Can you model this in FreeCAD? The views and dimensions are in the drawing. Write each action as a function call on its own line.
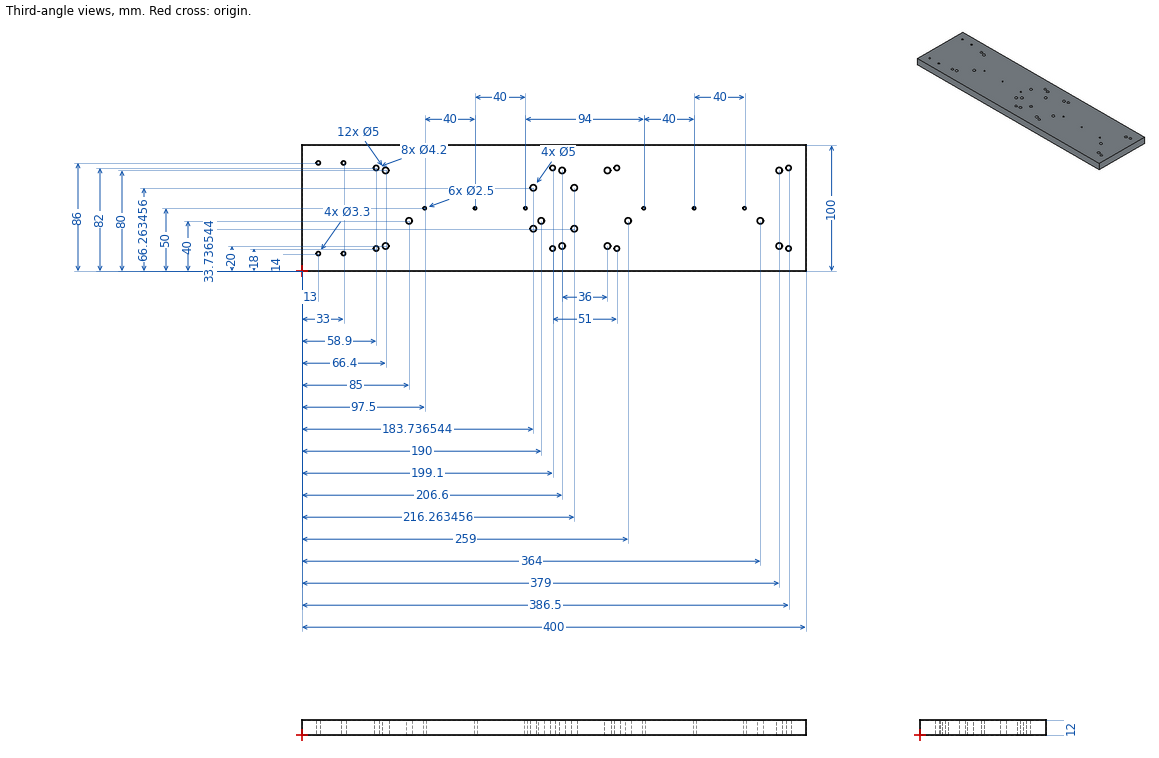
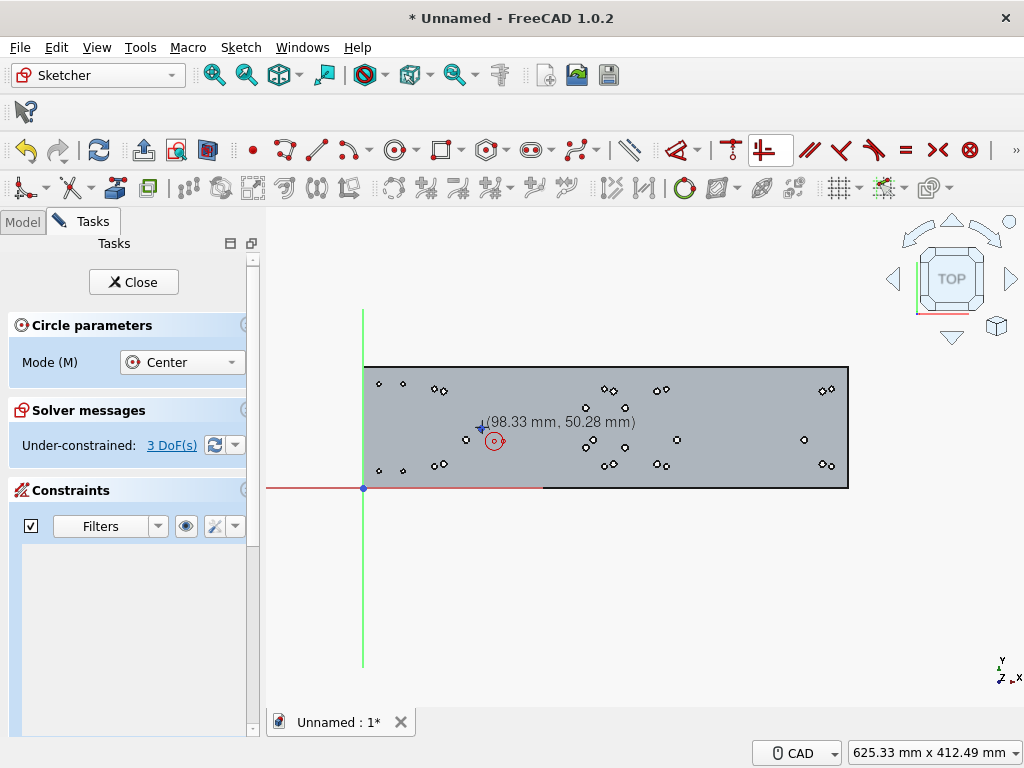
scroll(530, 428, up, 14)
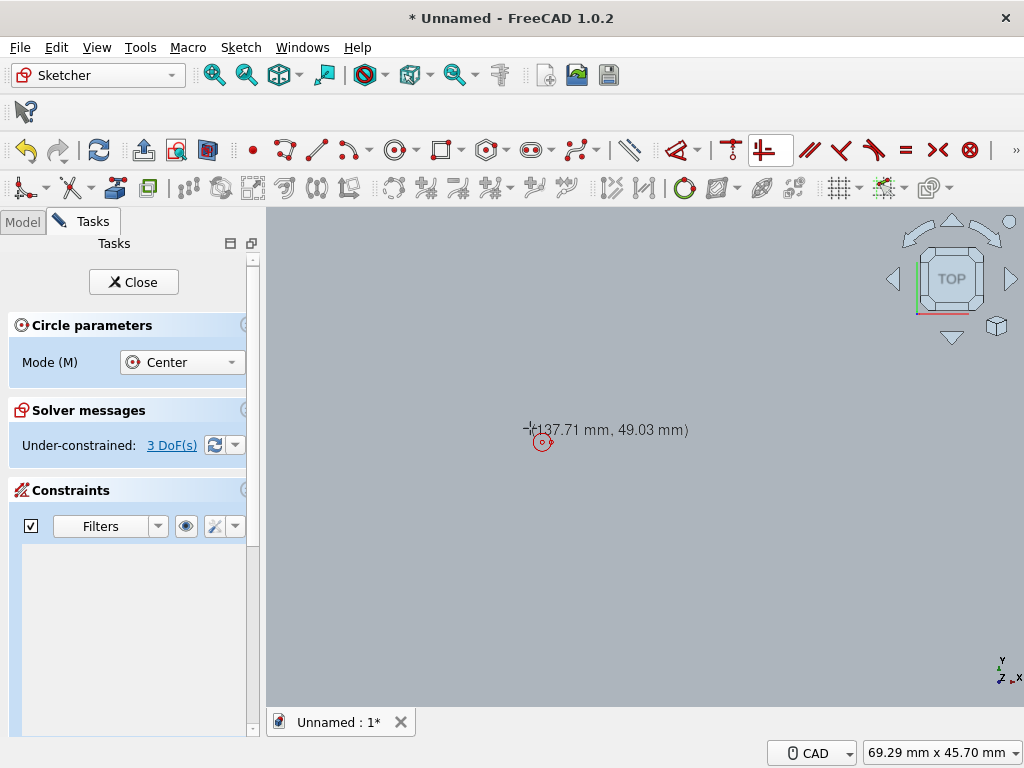
scroll(530, 428, down, 14)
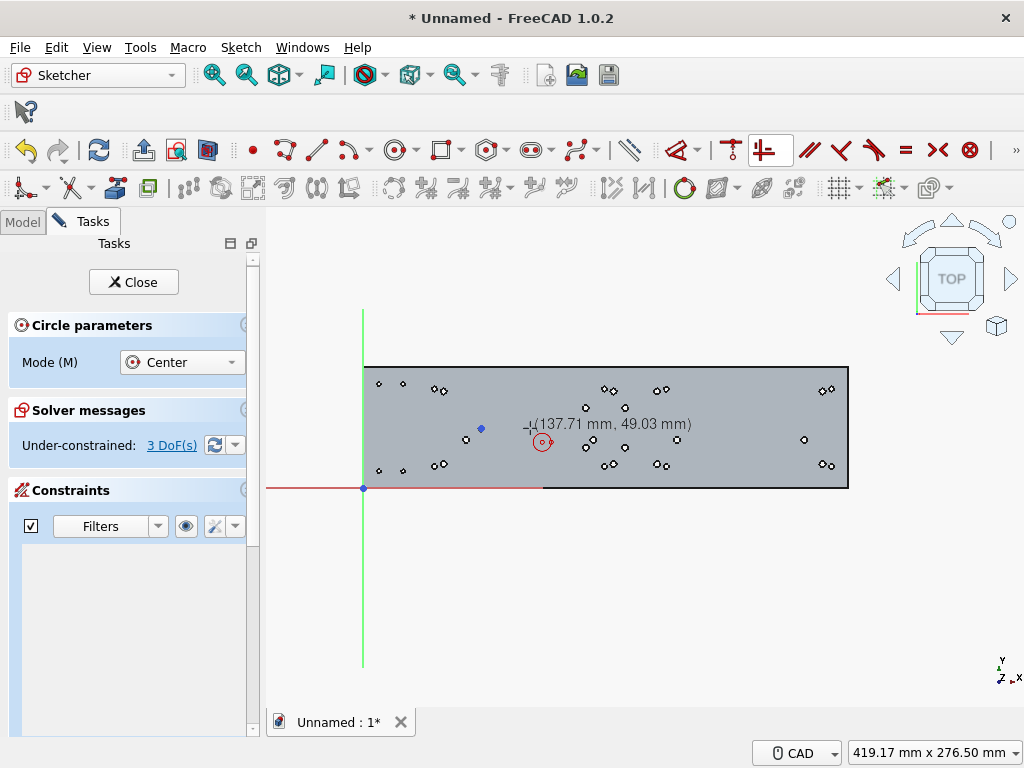
click(530, 428)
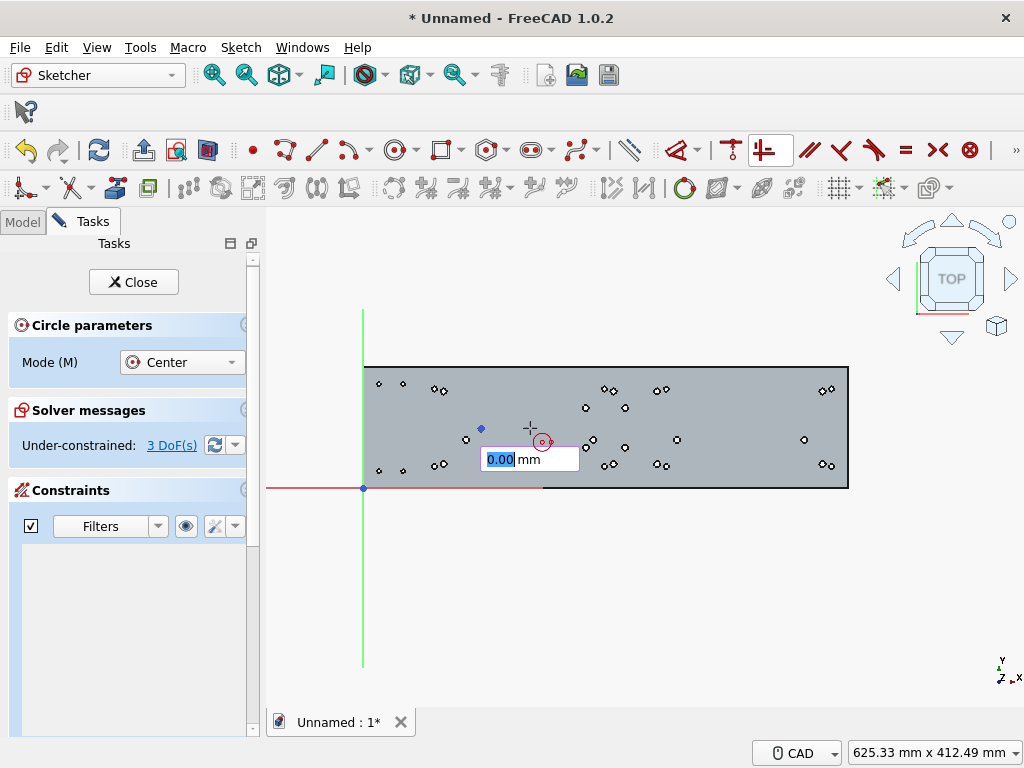
scroll(531, 427, up, 12)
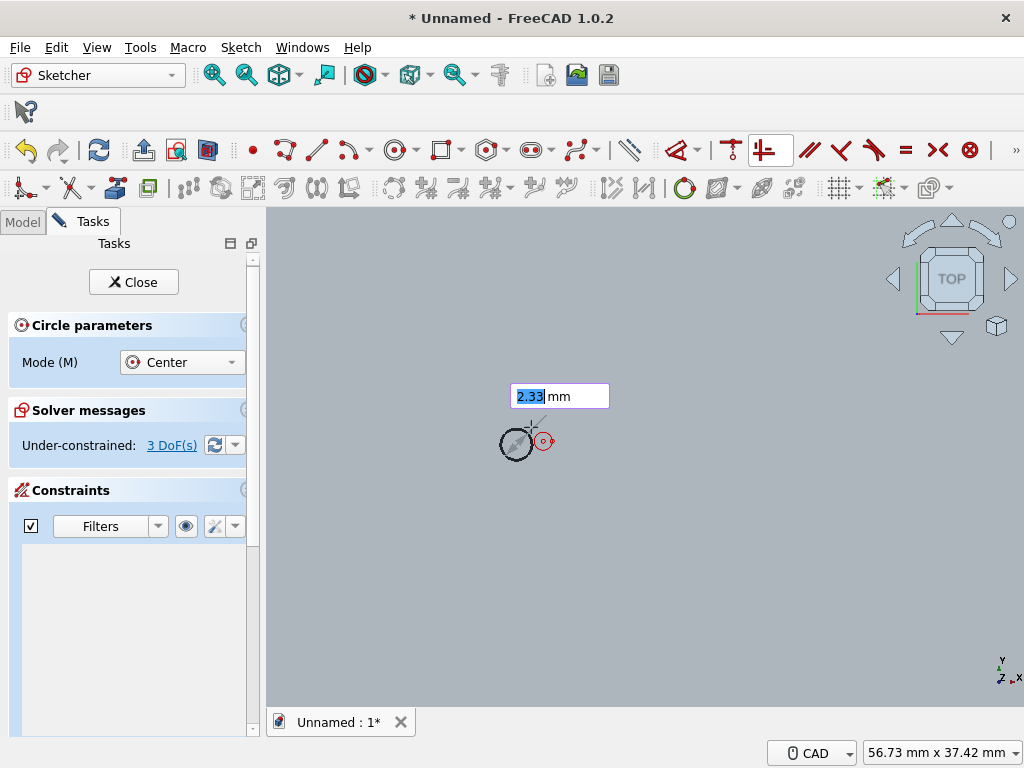
click(525, 420)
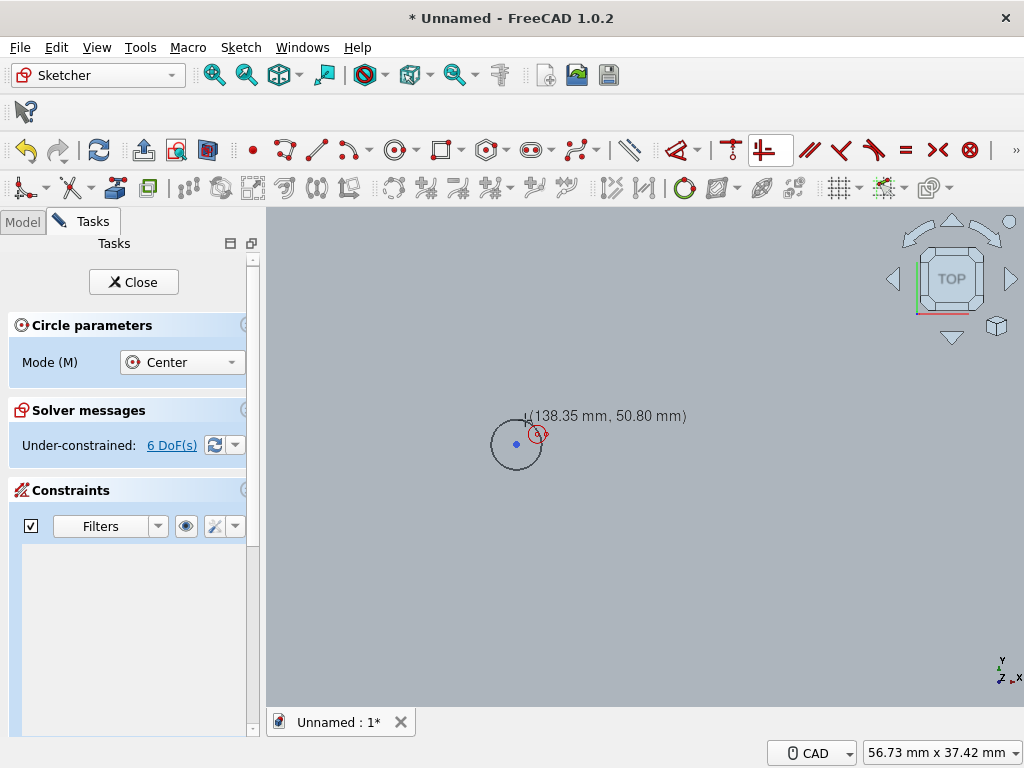
scroll(531, 427, down, 12)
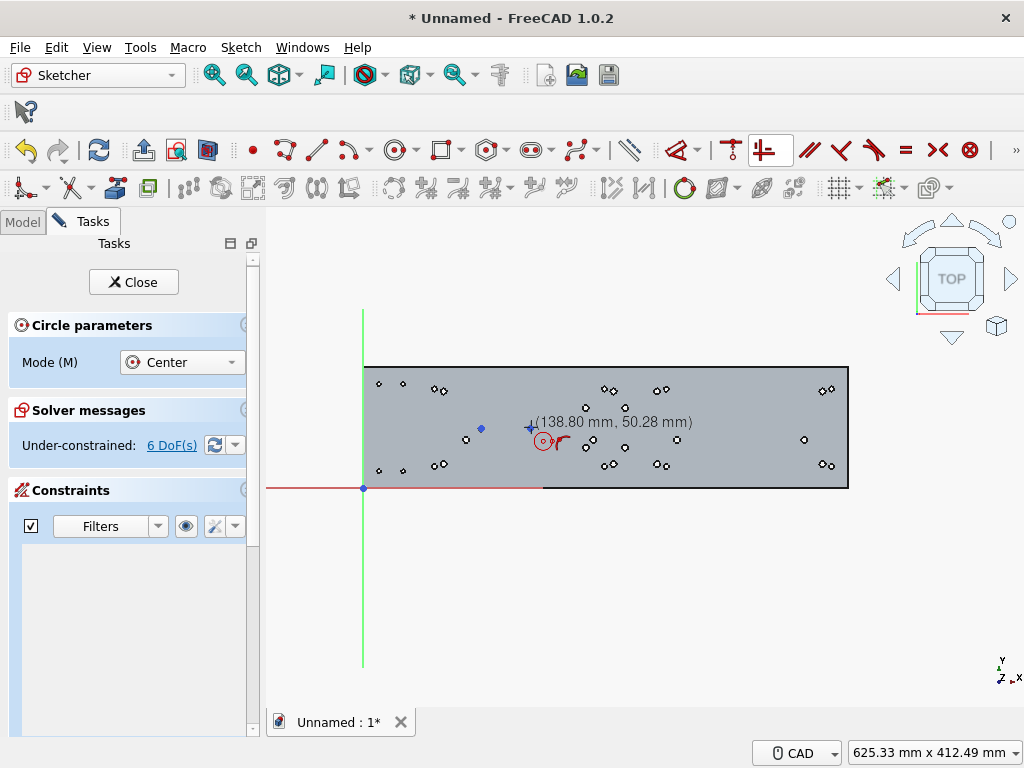
scroll(578, 428, up, 14)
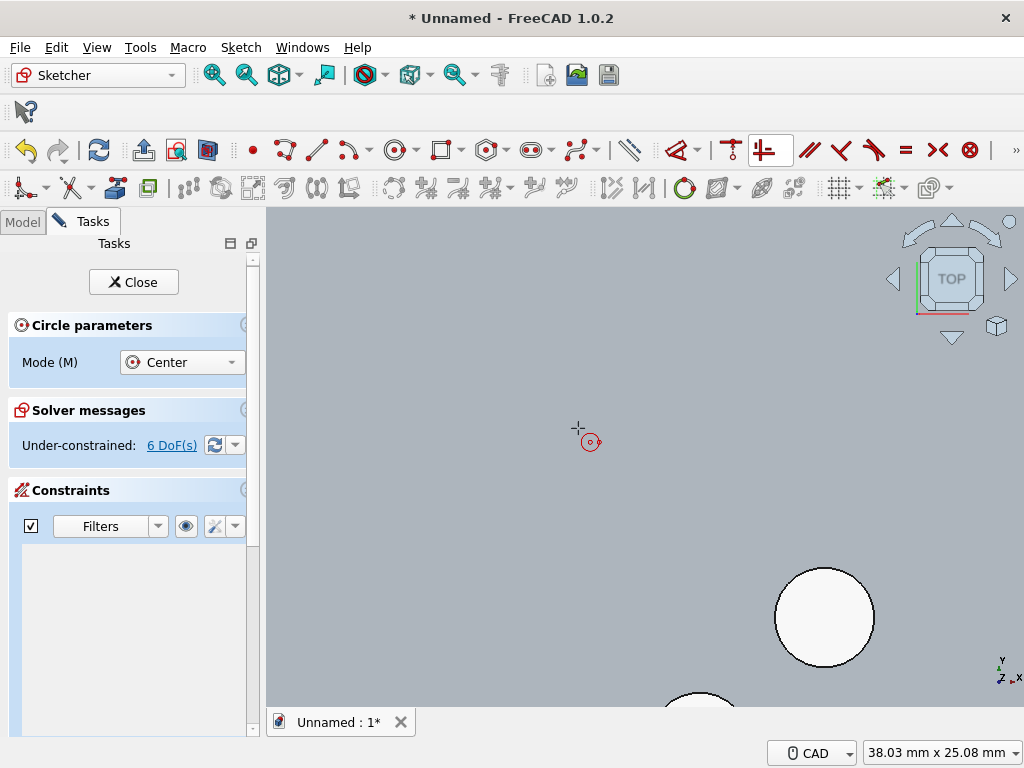
scroll(578, 428, down, 14)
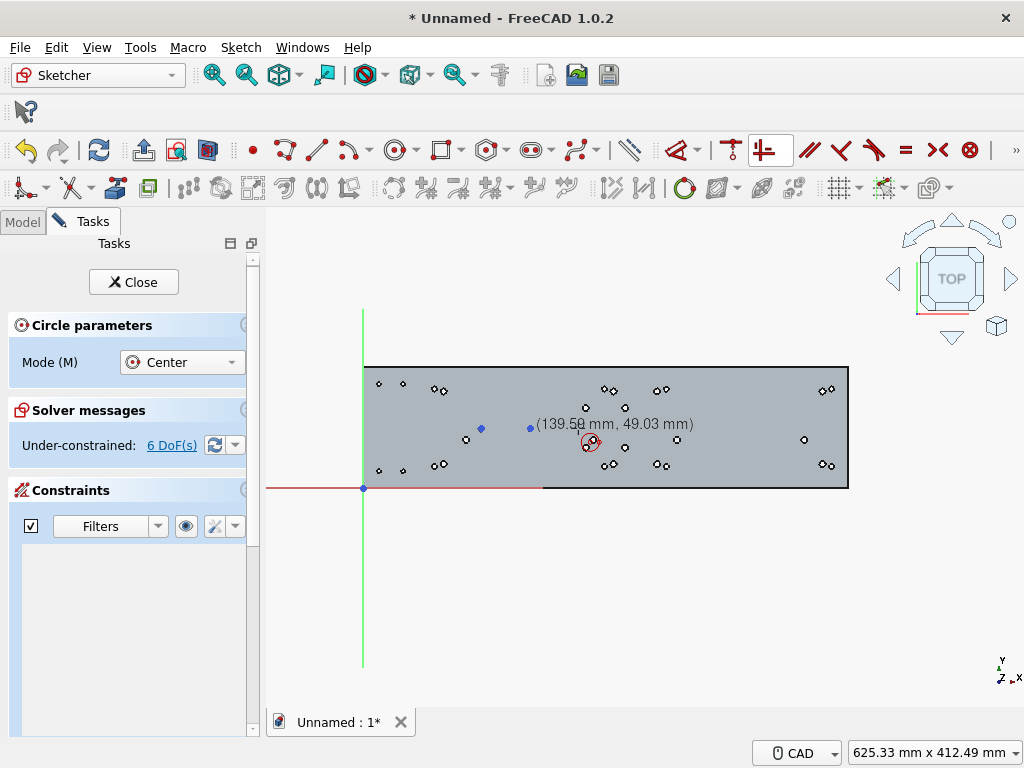
click(578, 428)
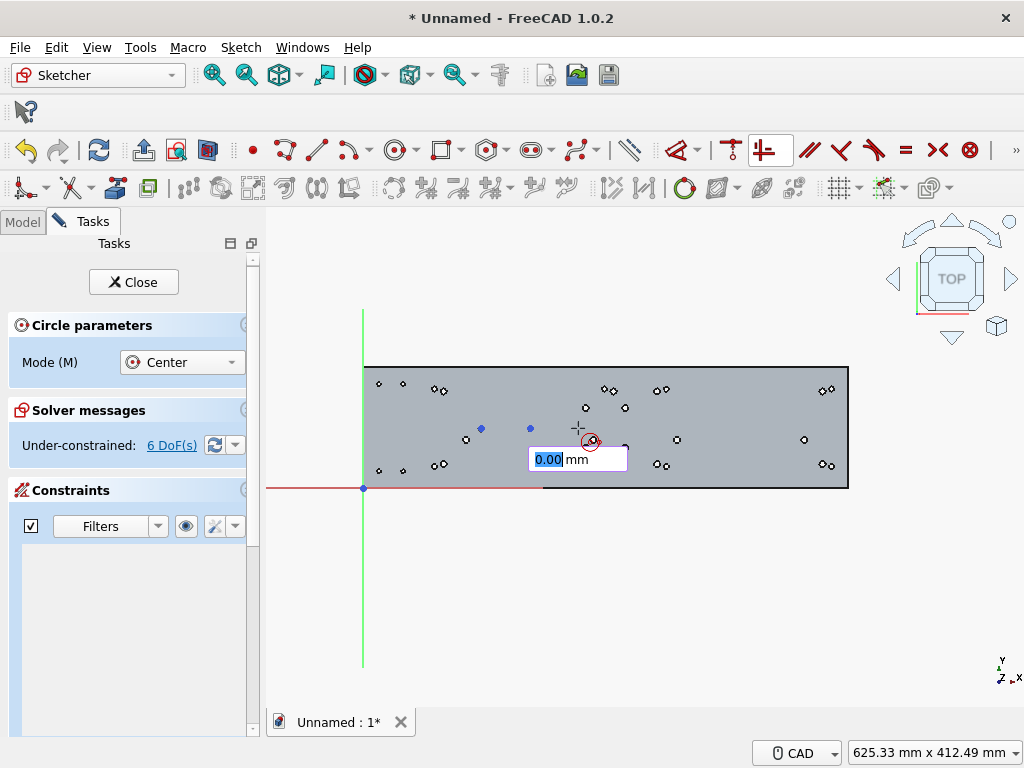
scroll(579, 427, up, 12)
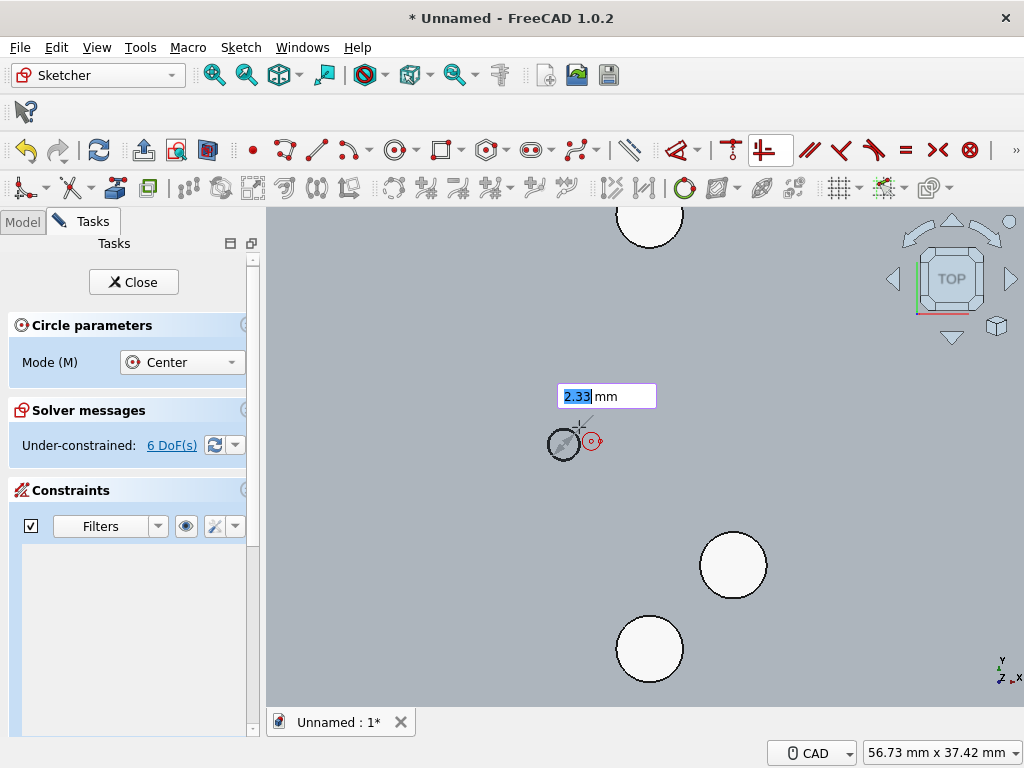
click(578, 420)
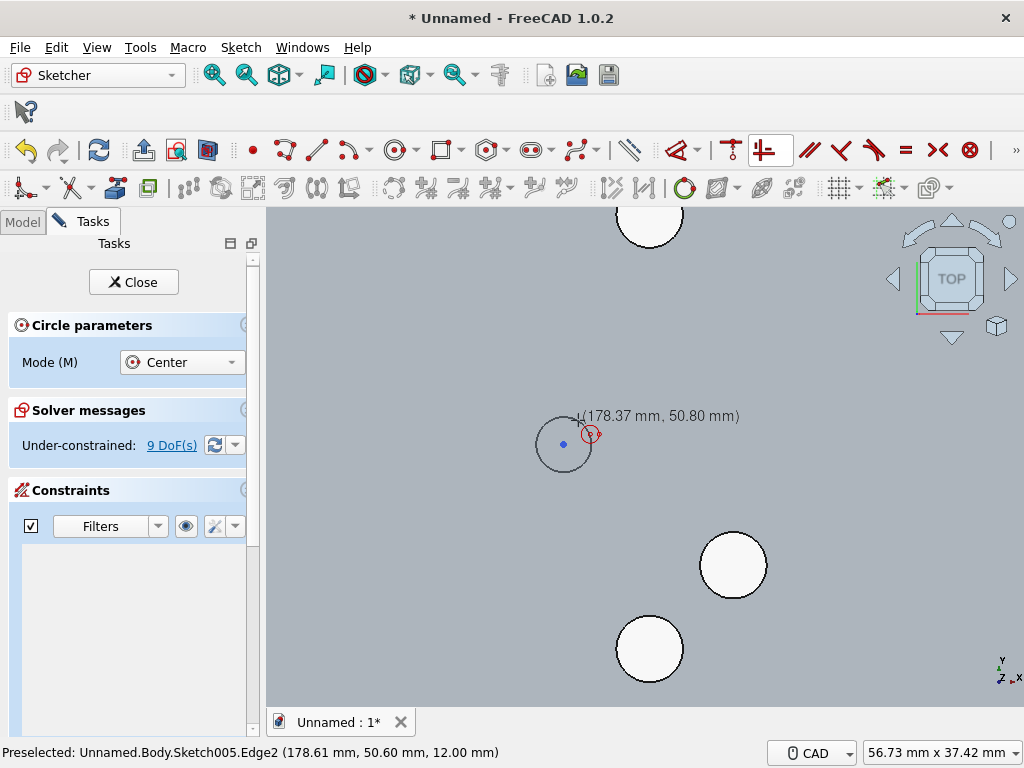
scroll(579, 427, down, 12)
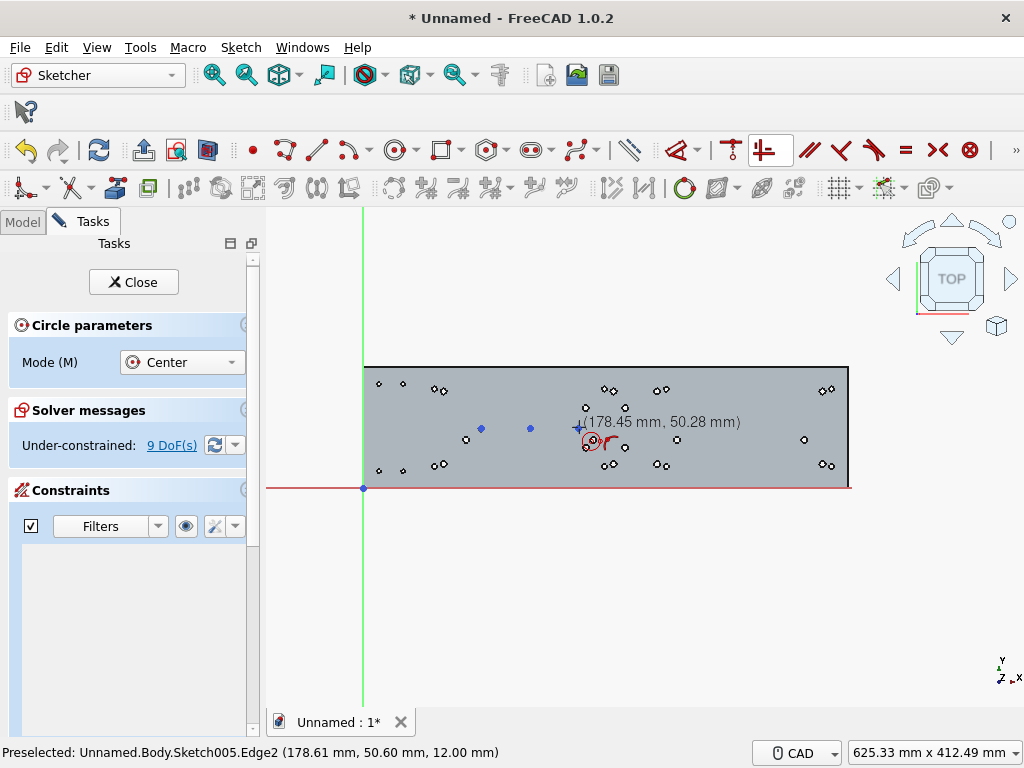
scroll(692, 428, up, 14)